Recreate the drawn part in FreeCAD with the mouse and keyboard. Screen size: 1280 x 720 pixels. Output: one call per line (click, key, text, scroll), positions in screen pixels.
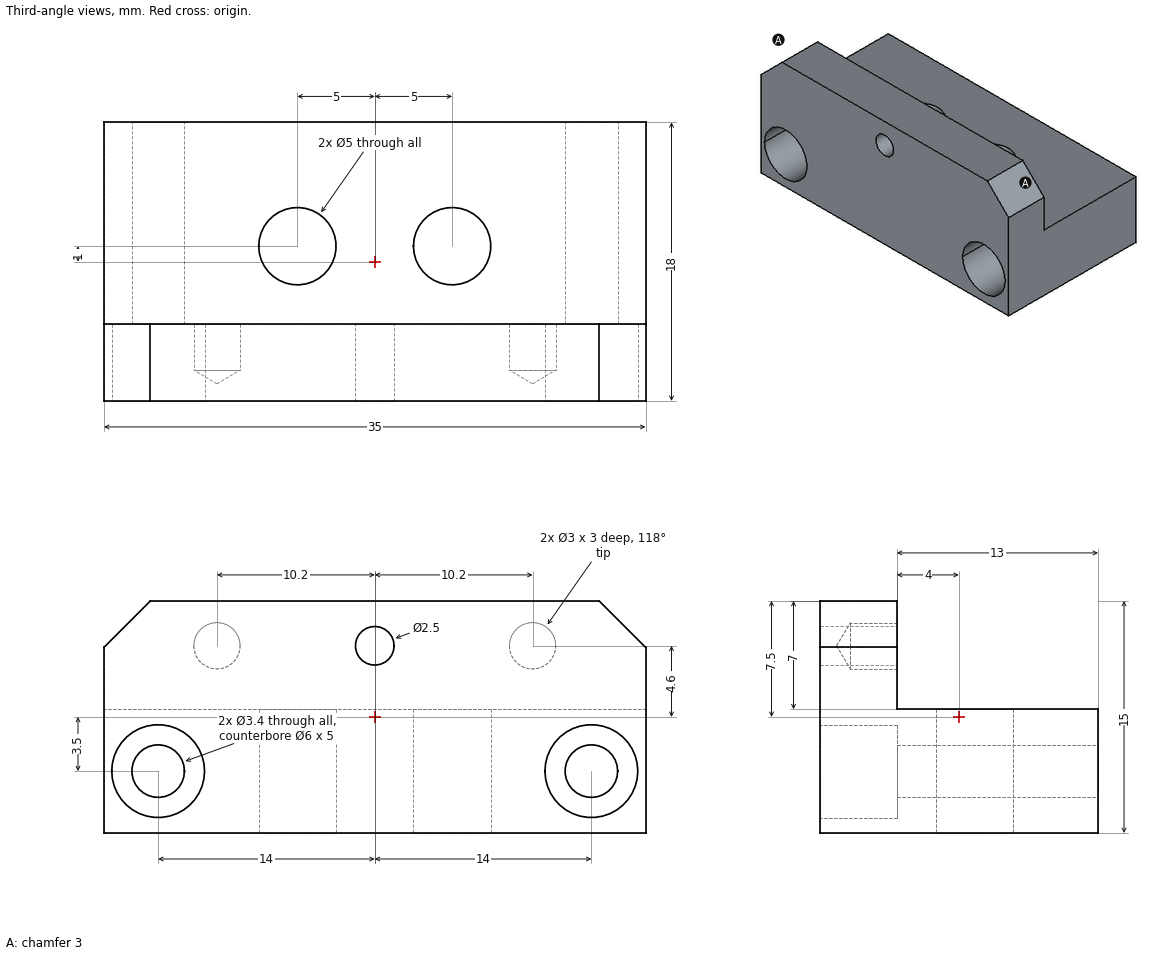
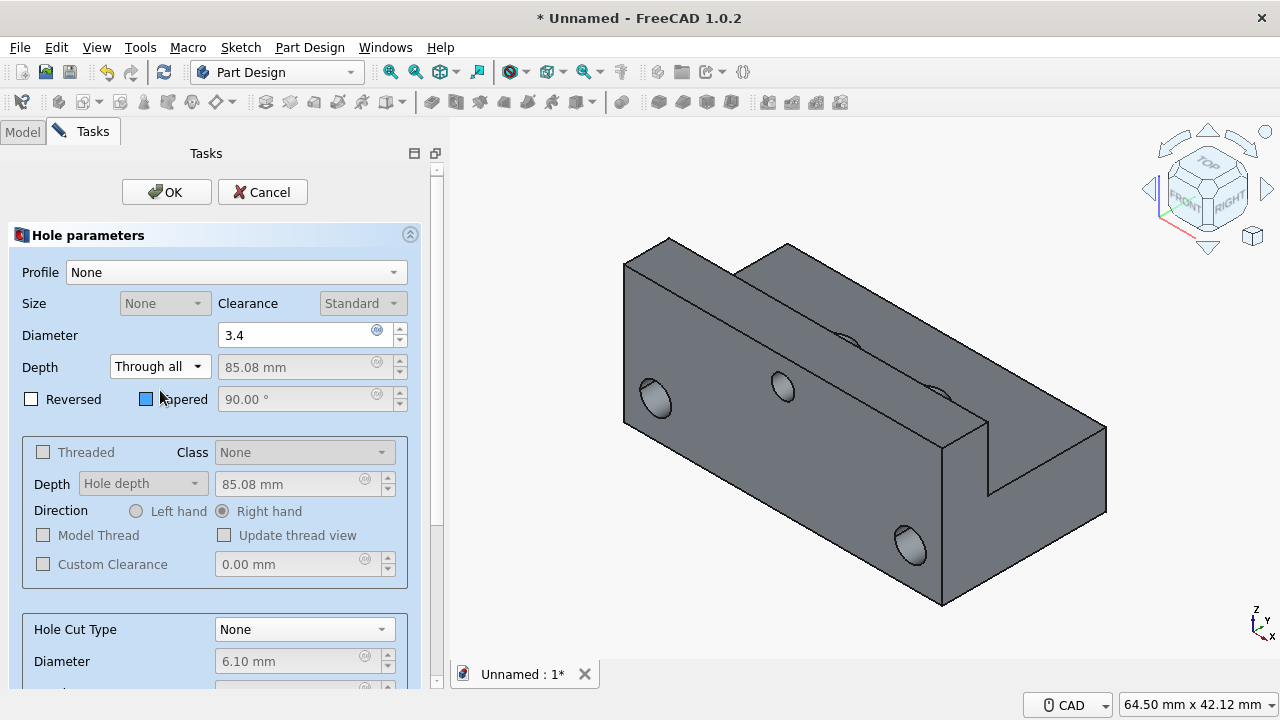
click(306, 630)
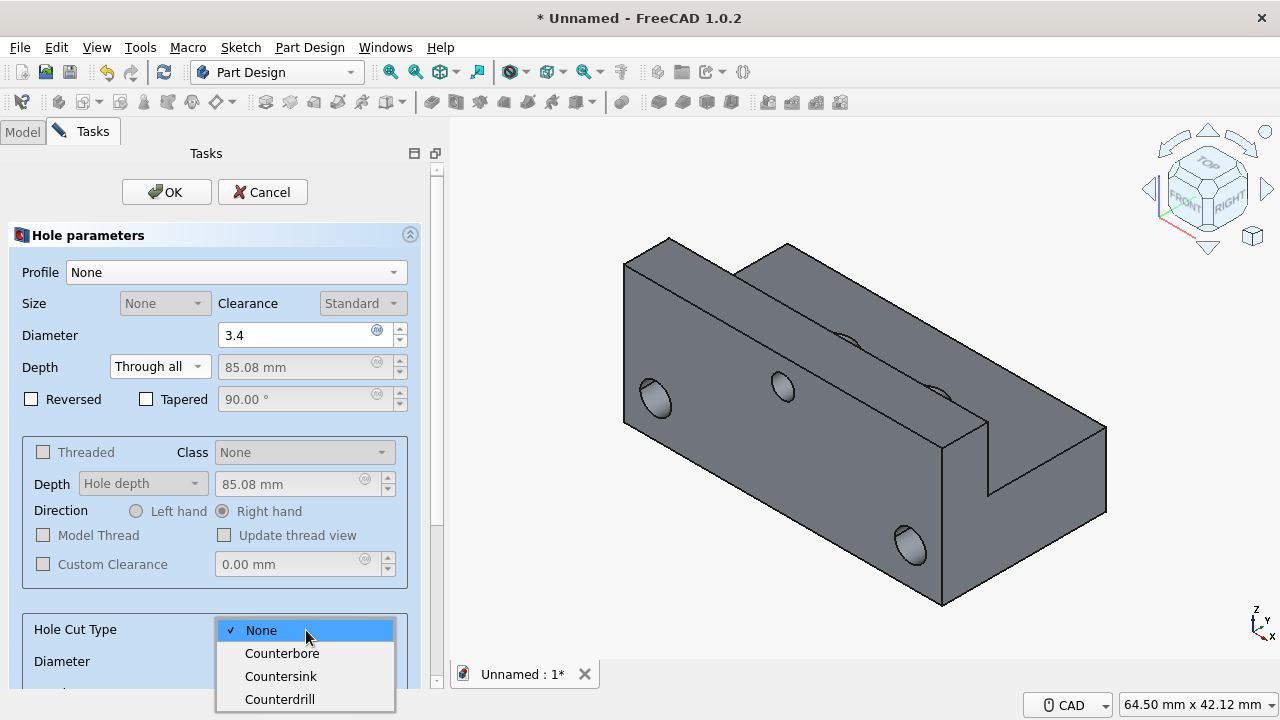
click(304, 654)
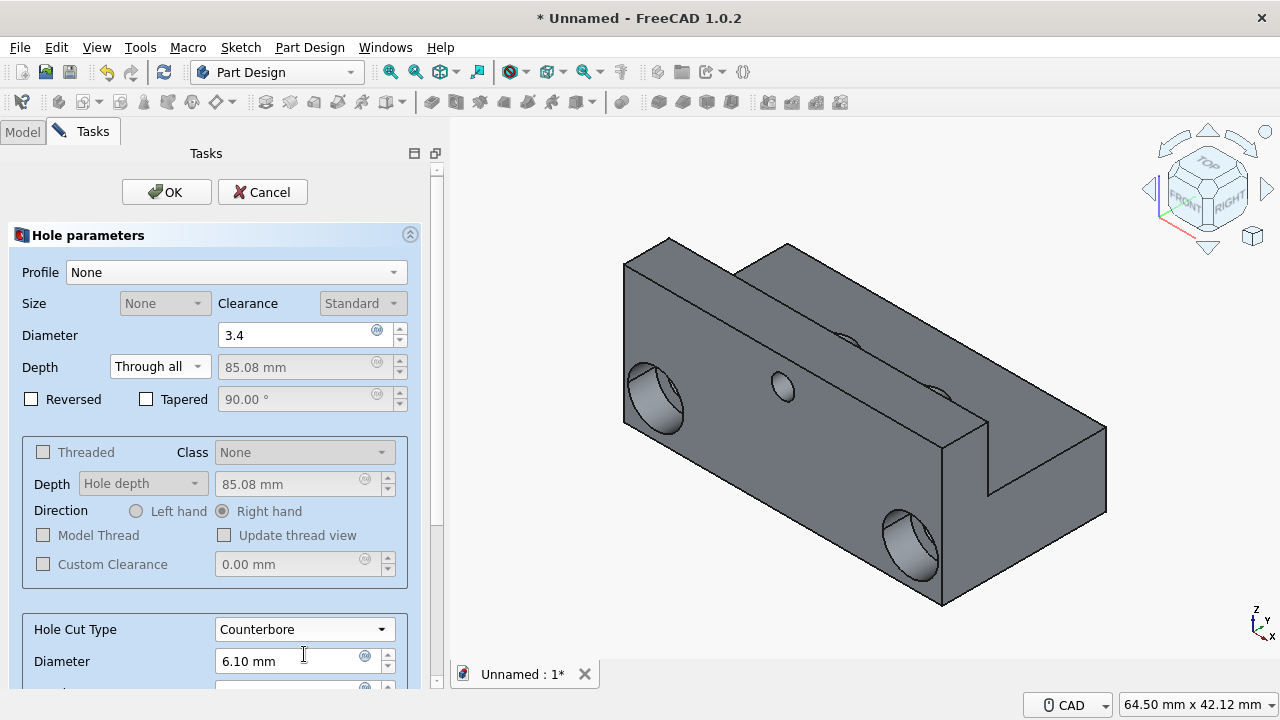
triple_click(298, 661)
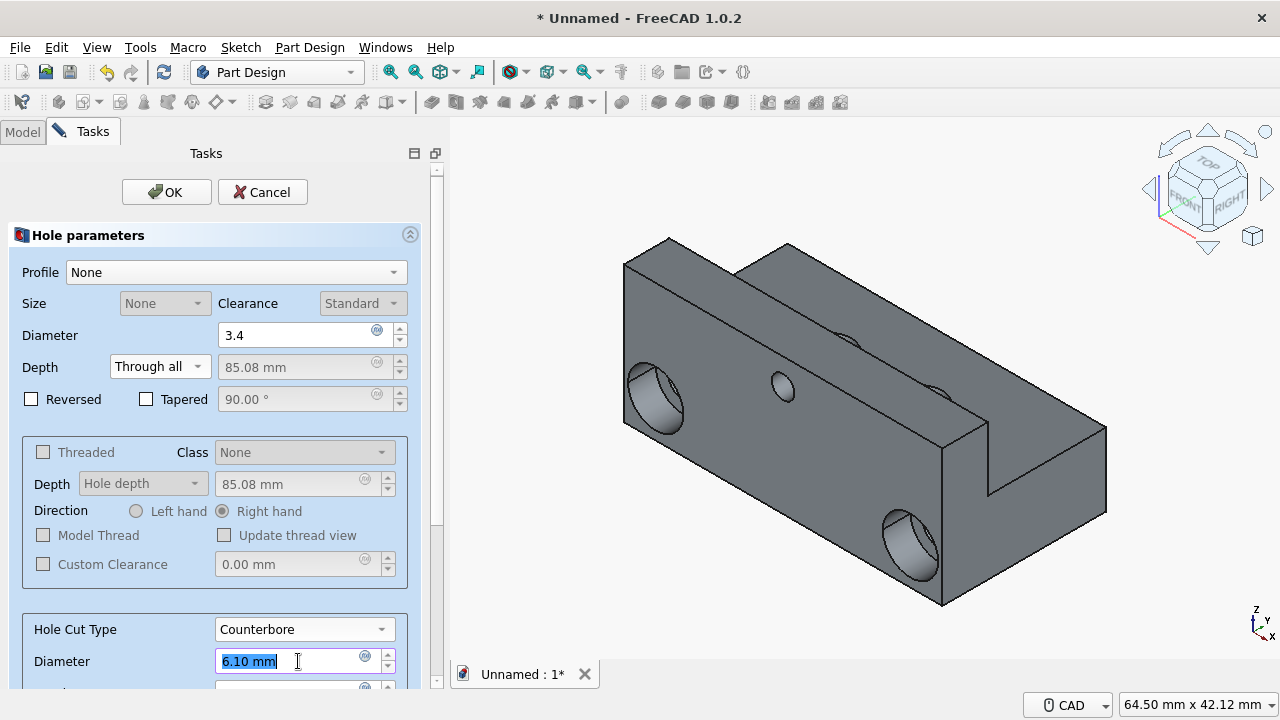
text(6)
key(Tab)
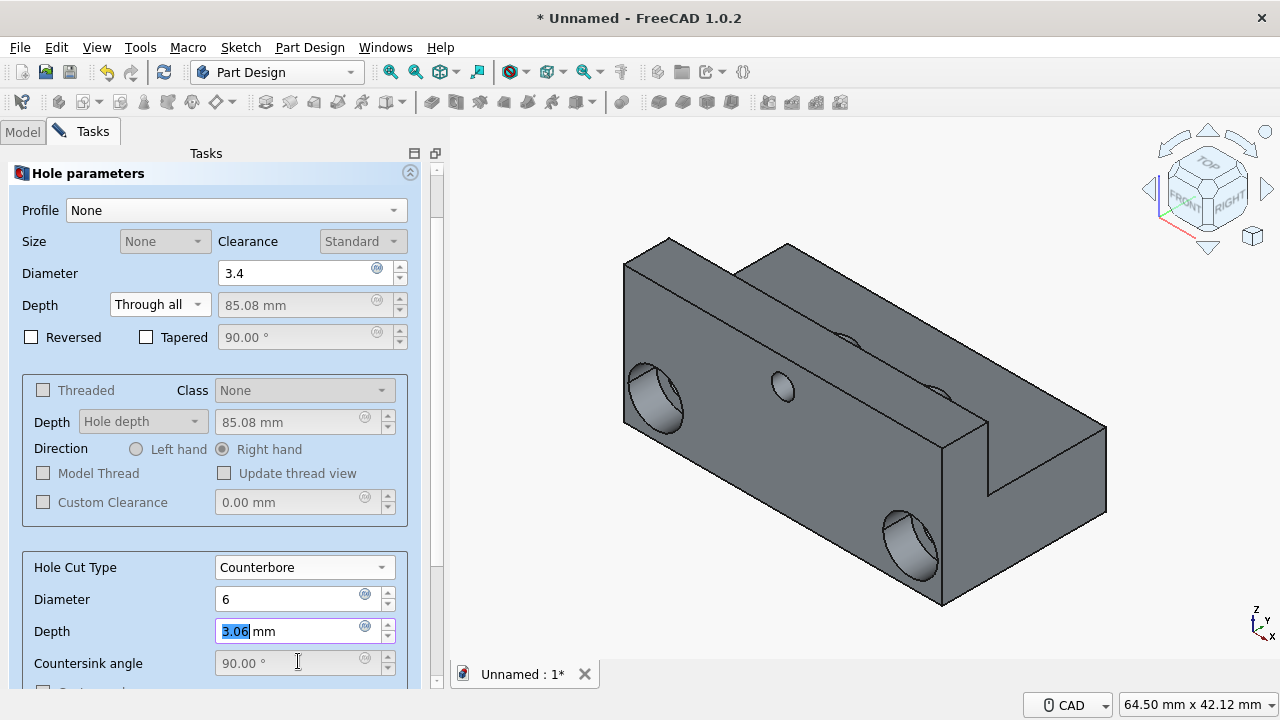
text(5)
key(Tab)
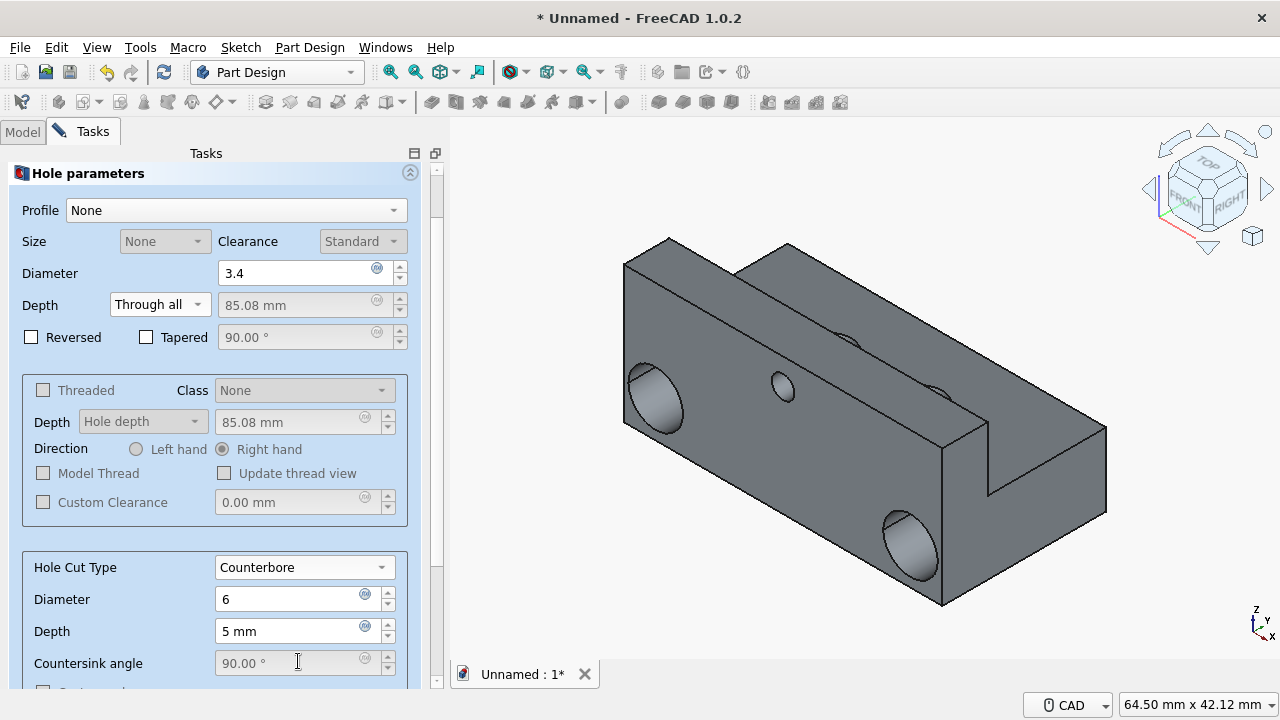
scroll(437, 426, up, 2)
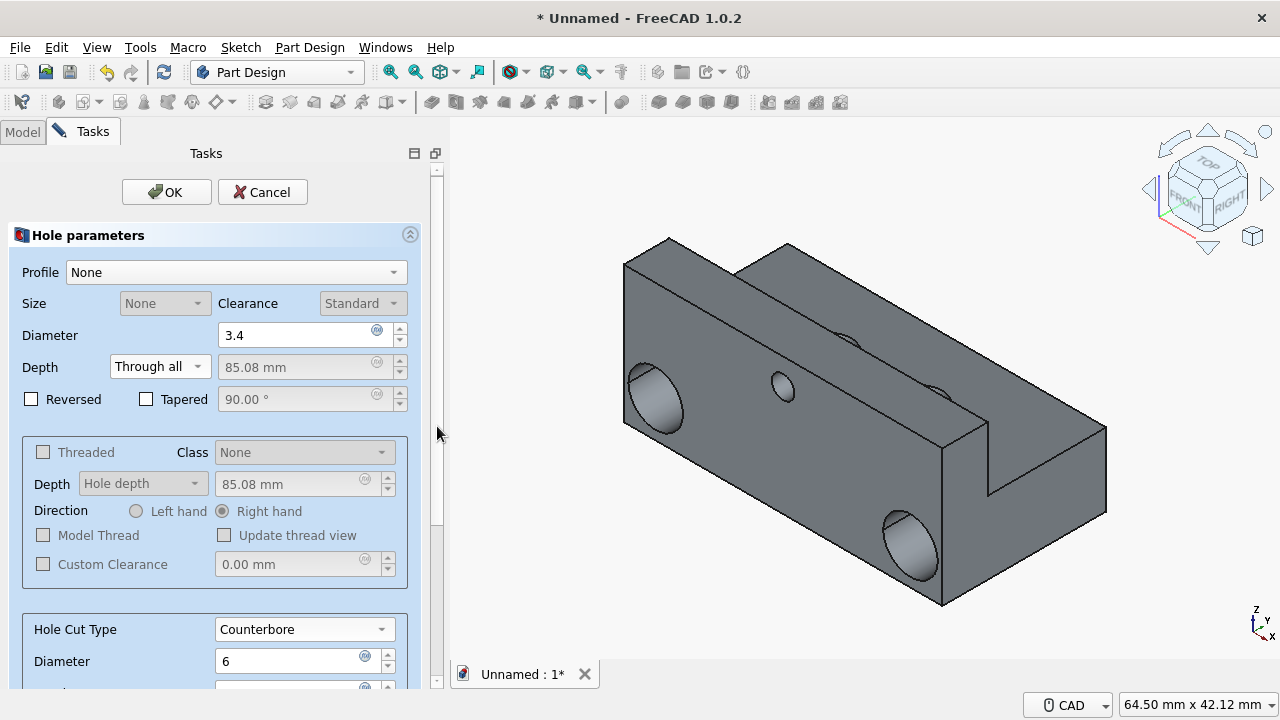
click(167, 192)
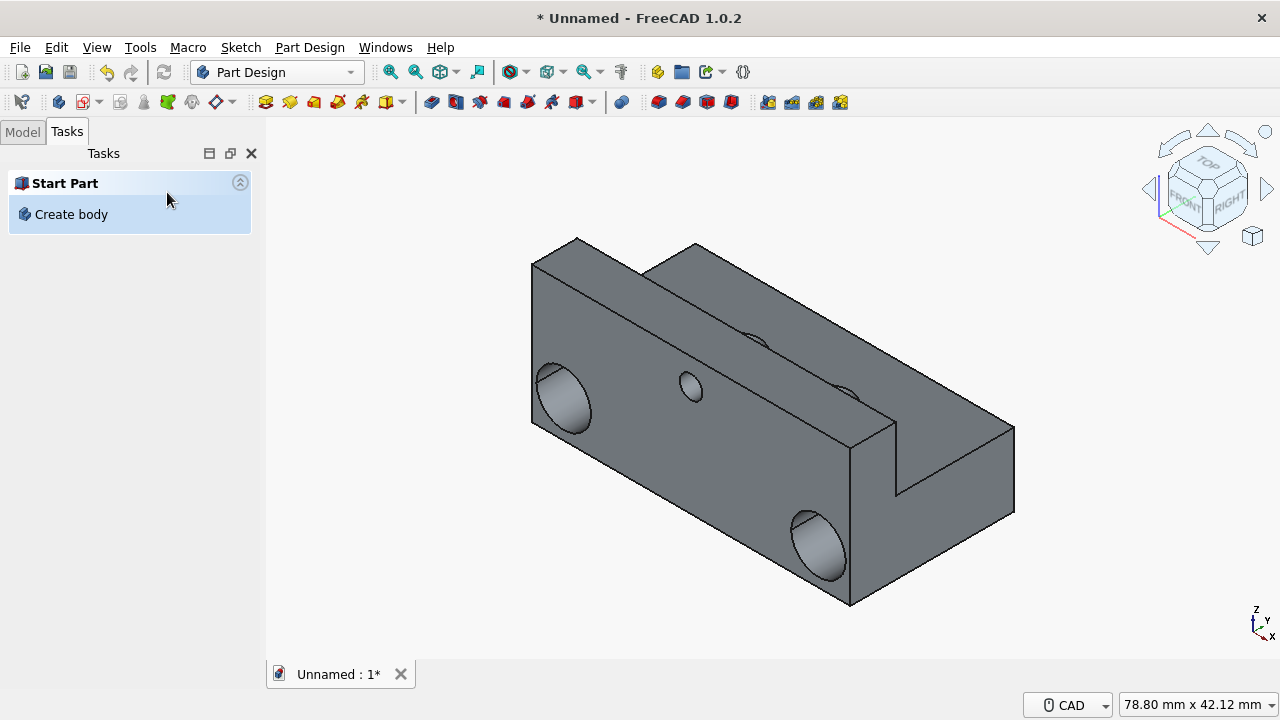
click(873, 434)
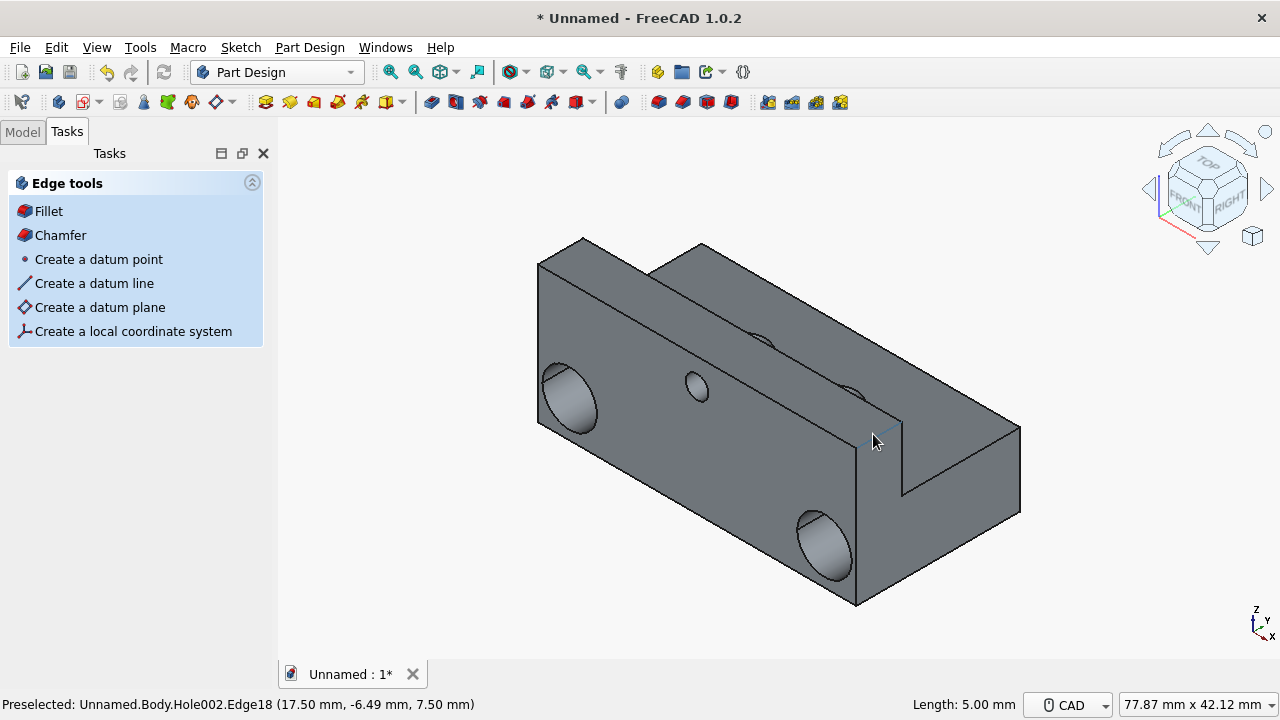
key(2)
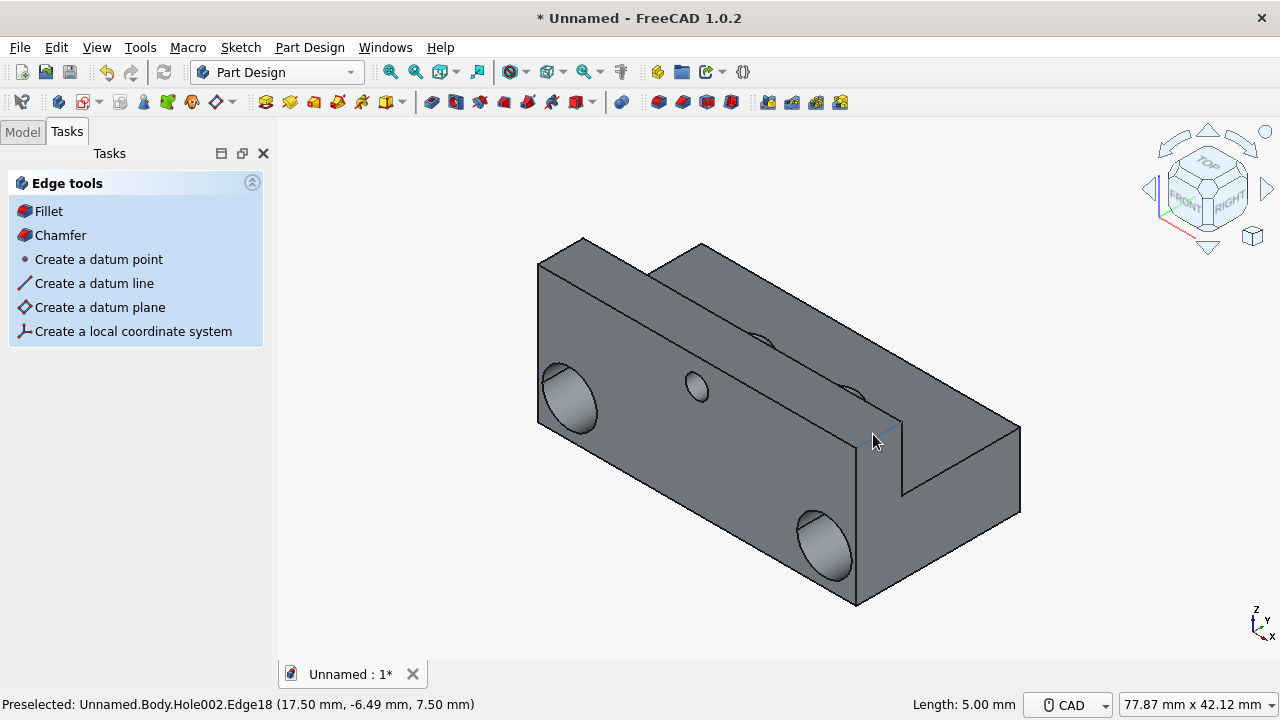
key(v)
key(f)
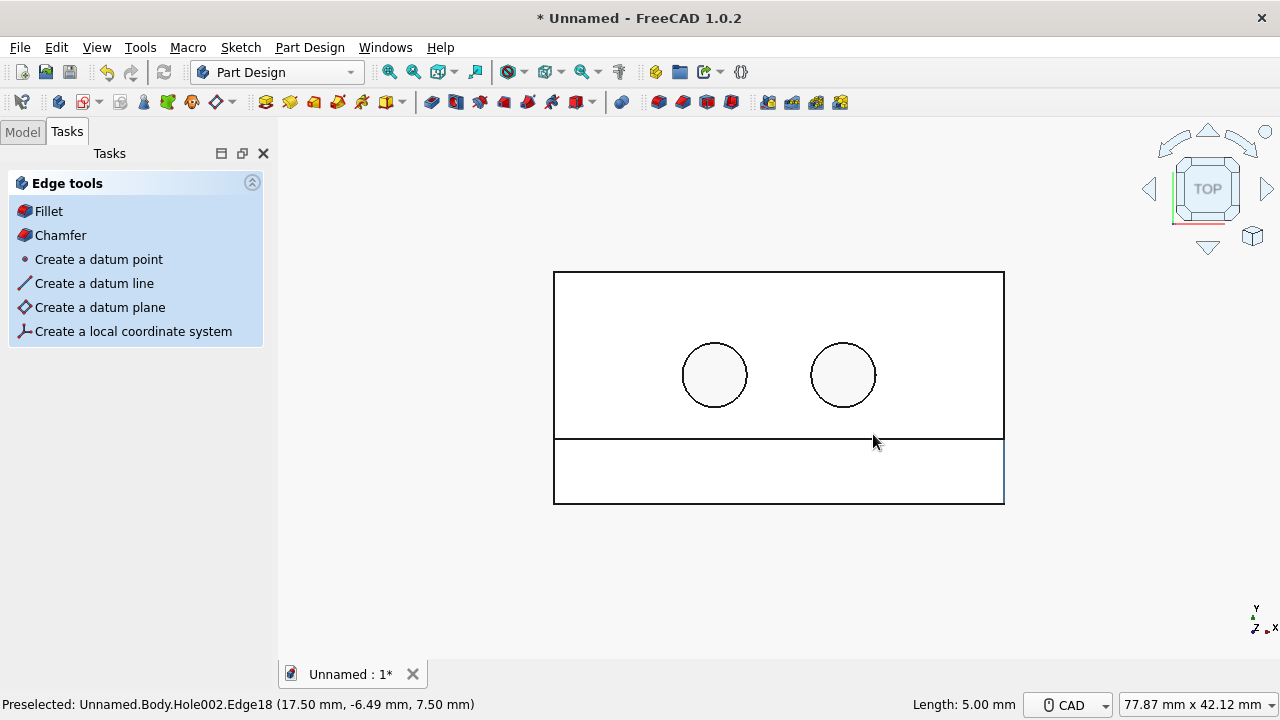
click(554, 471, ctrl)